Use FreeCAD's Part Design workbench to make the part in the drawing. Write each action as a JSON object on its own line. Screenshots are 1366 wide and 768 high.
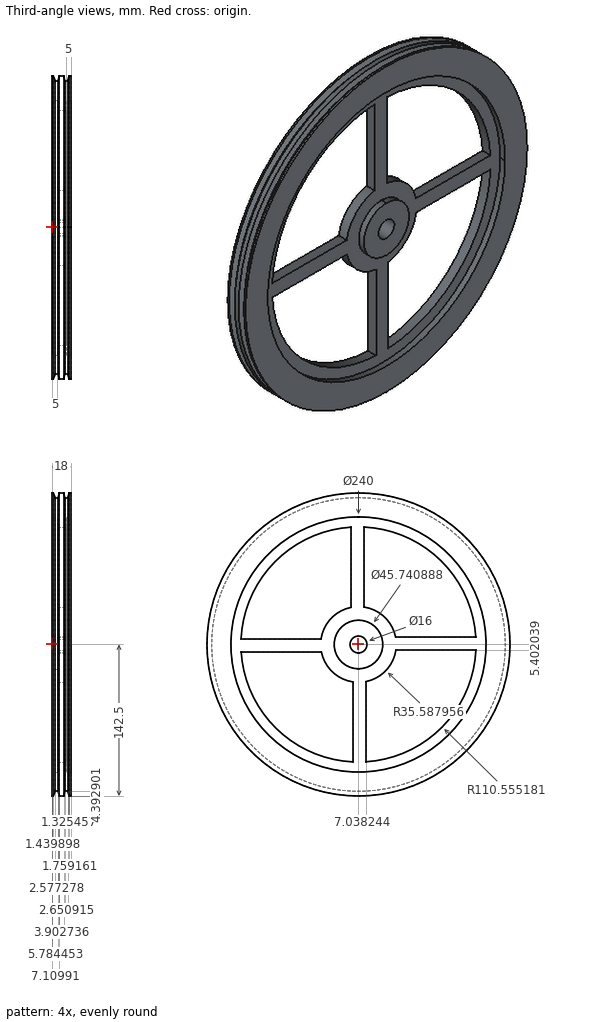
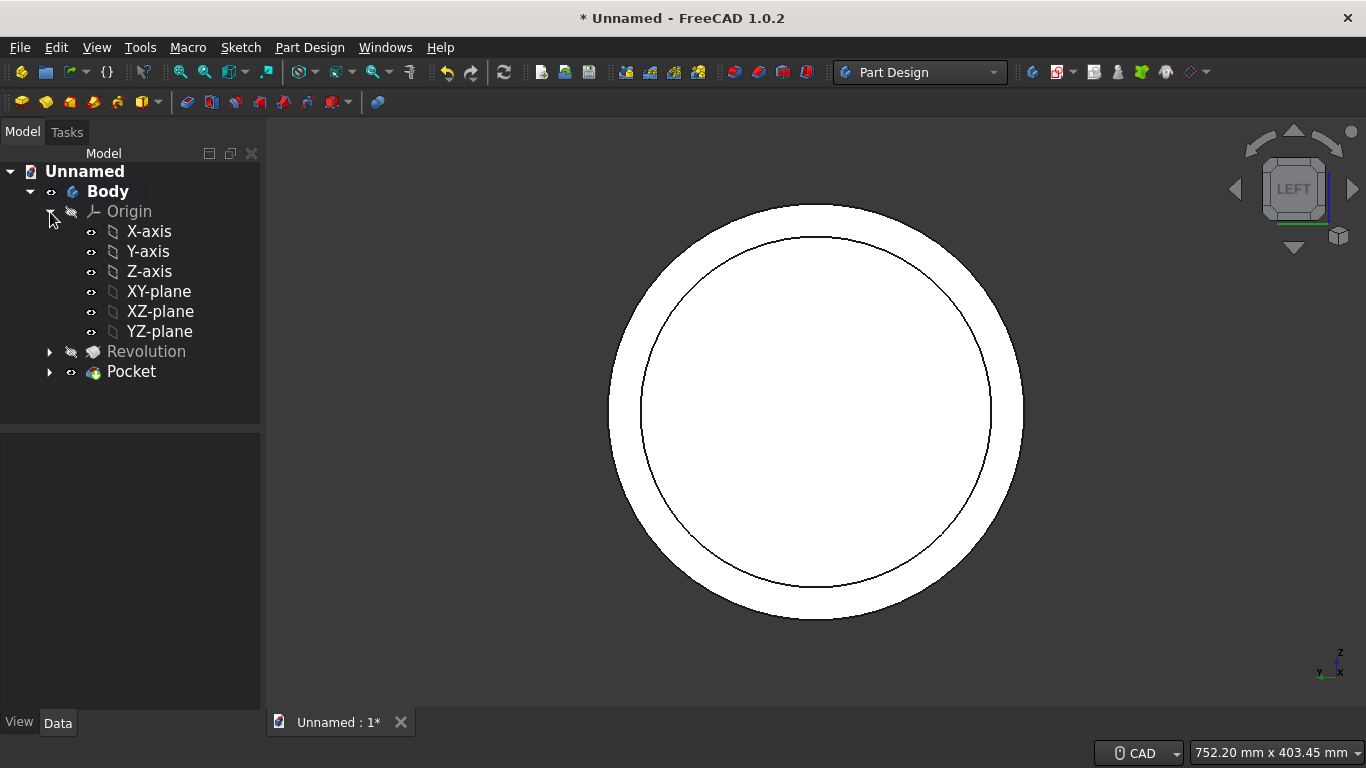
{"action": "left_click", "coordinate": [136, 332]}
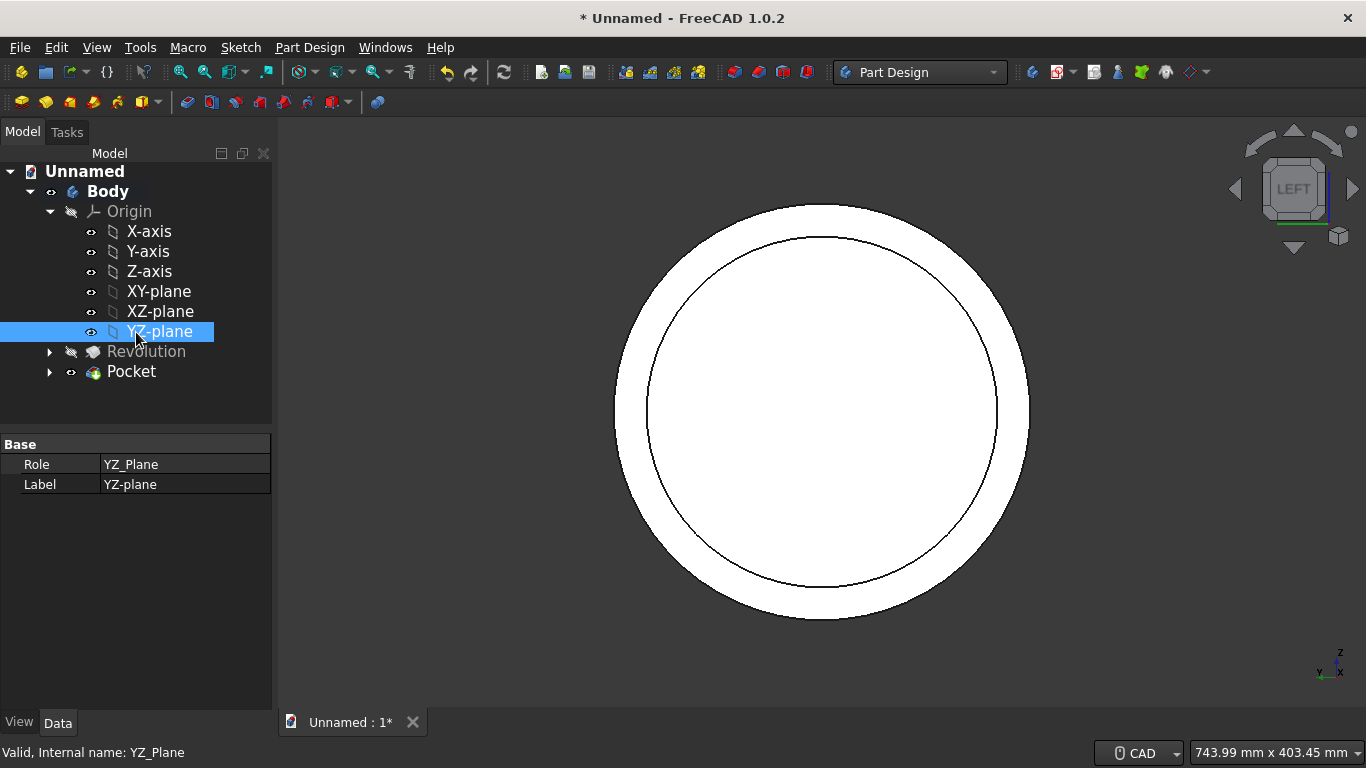
{"action": "left_click", "coordinate": [1190, 72]}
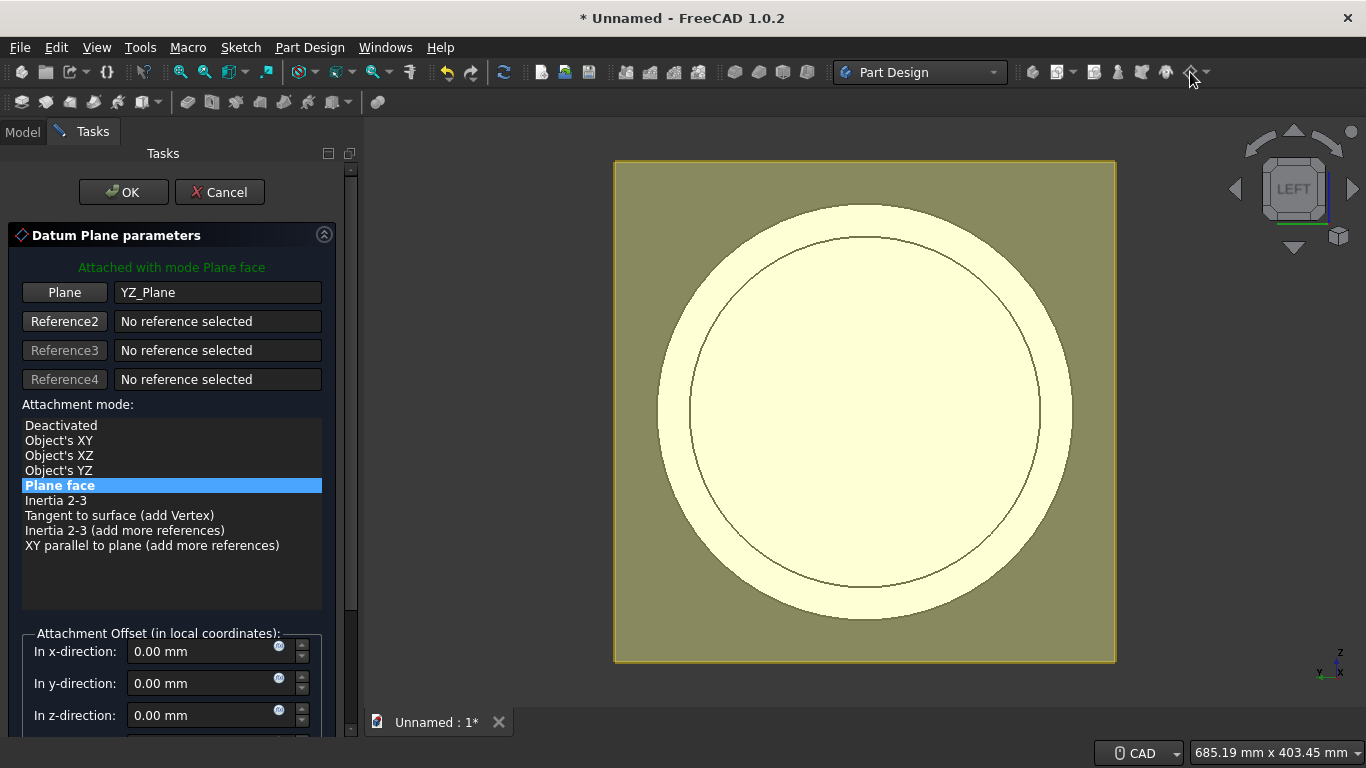
{"action": "triple_click", "coordinate": [210, 715]}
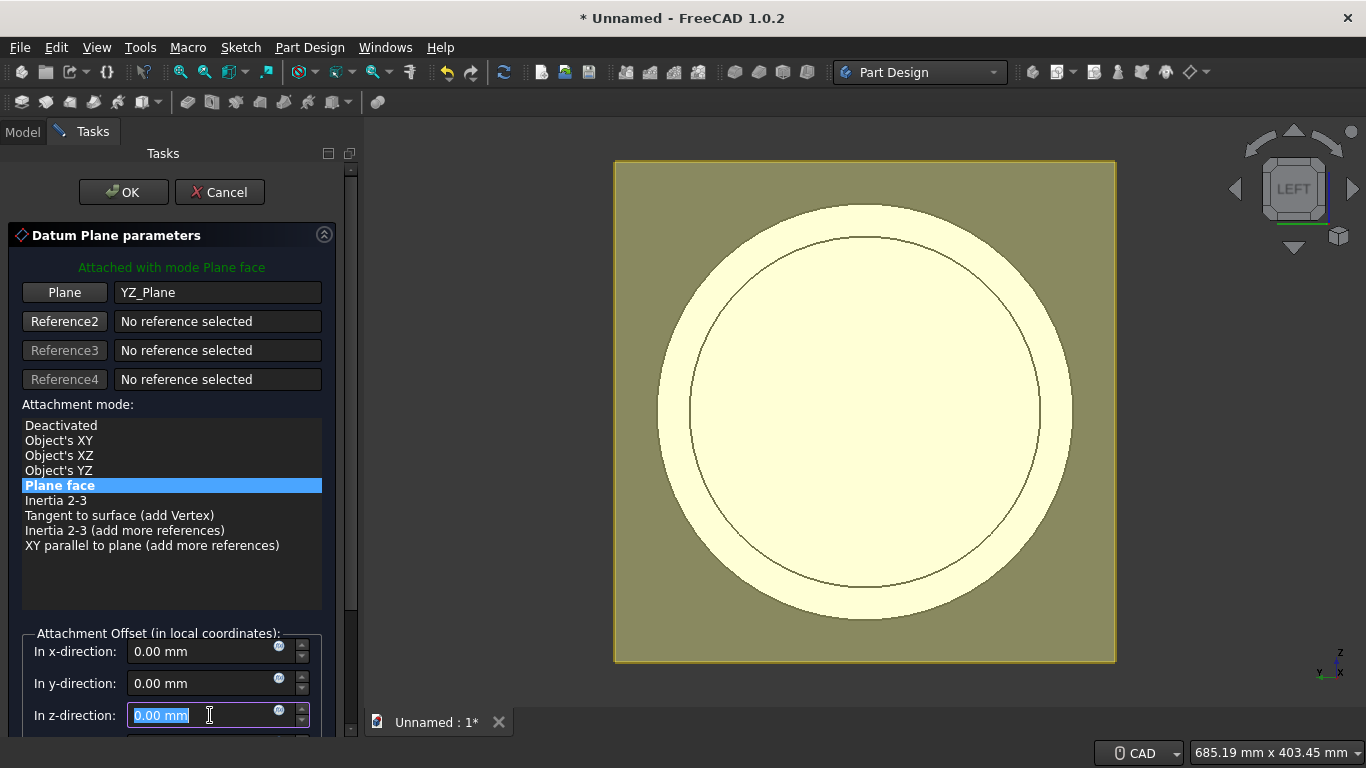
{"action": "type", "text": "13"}
{"action": "key", "text": "Tab"}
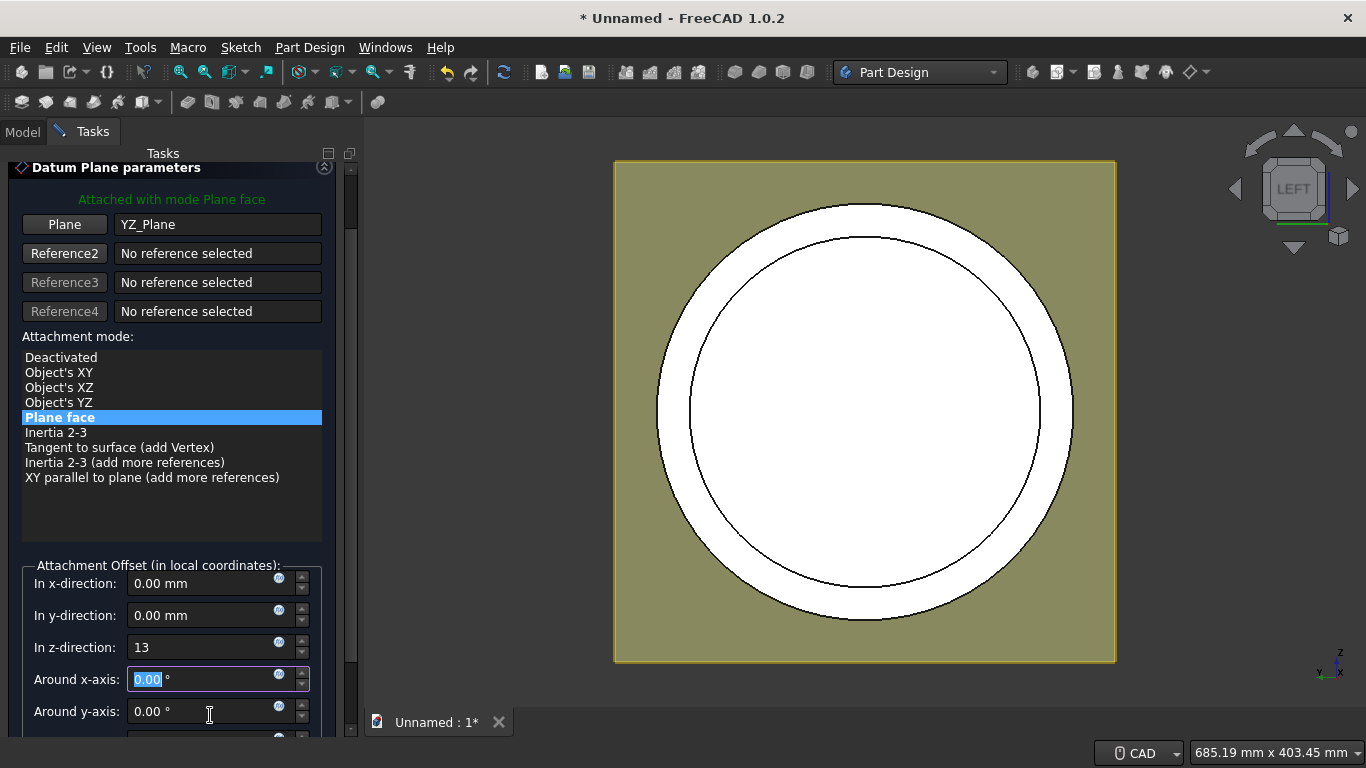
{"action": "scroll", "coordinate": [351, 450], "scroll_direction": "up", "scroll_amount": 2}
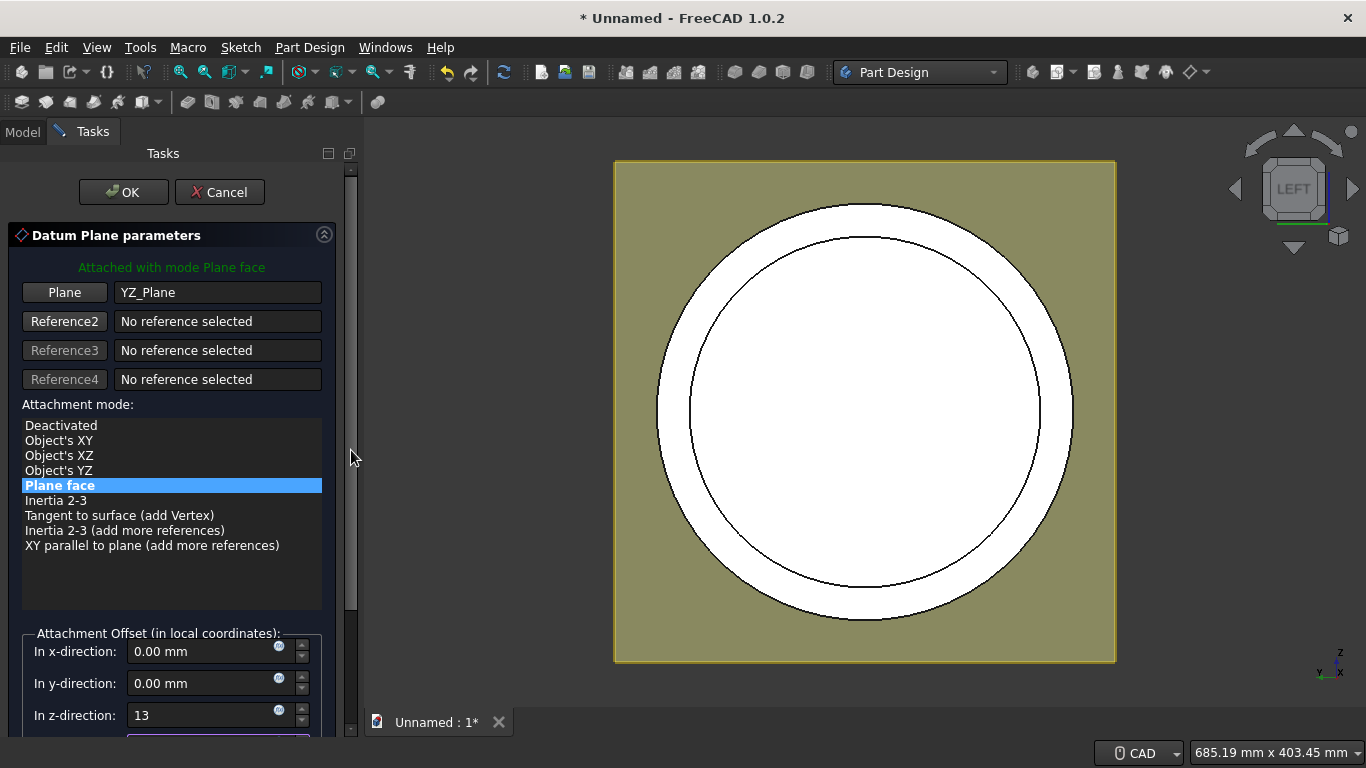
{"action": "left_click", "coordinate": [124, 192]}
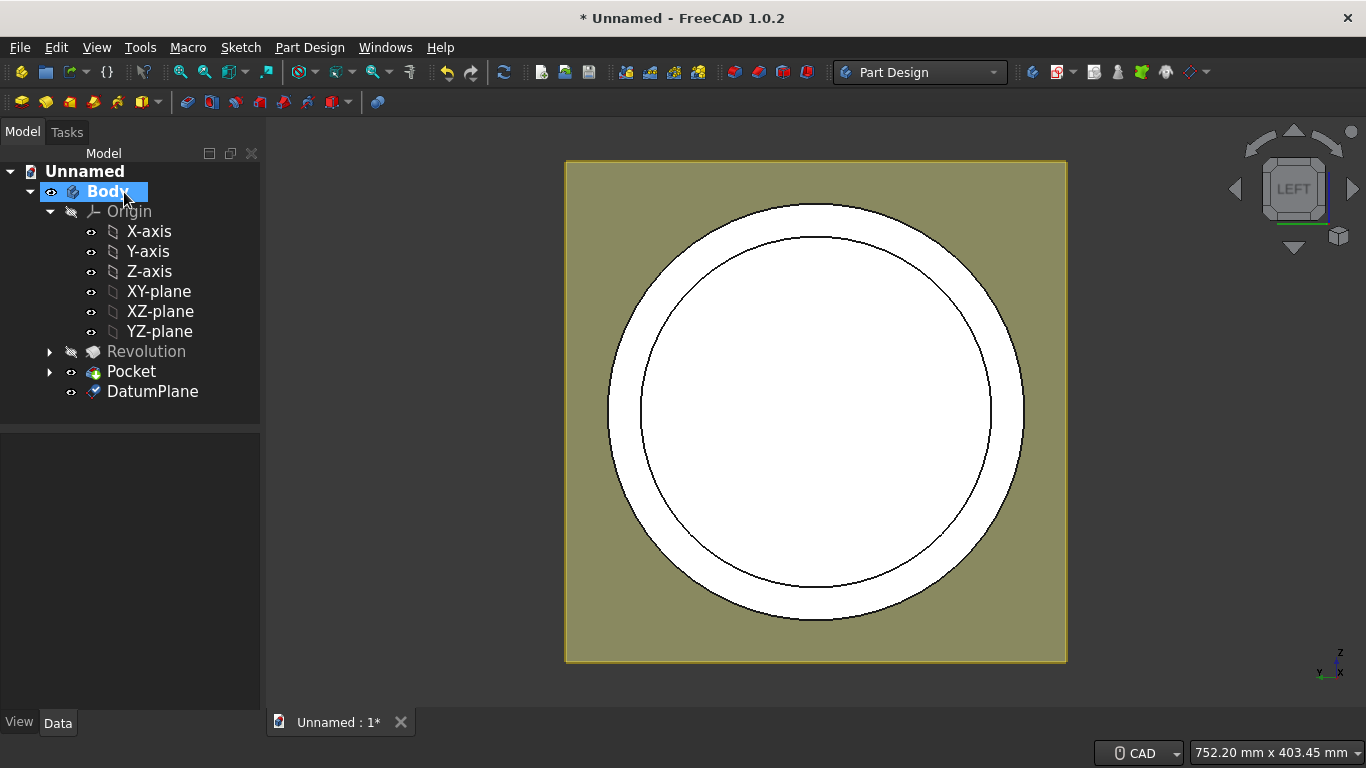
{"action": "left_click", "coordinate": [116, 392]}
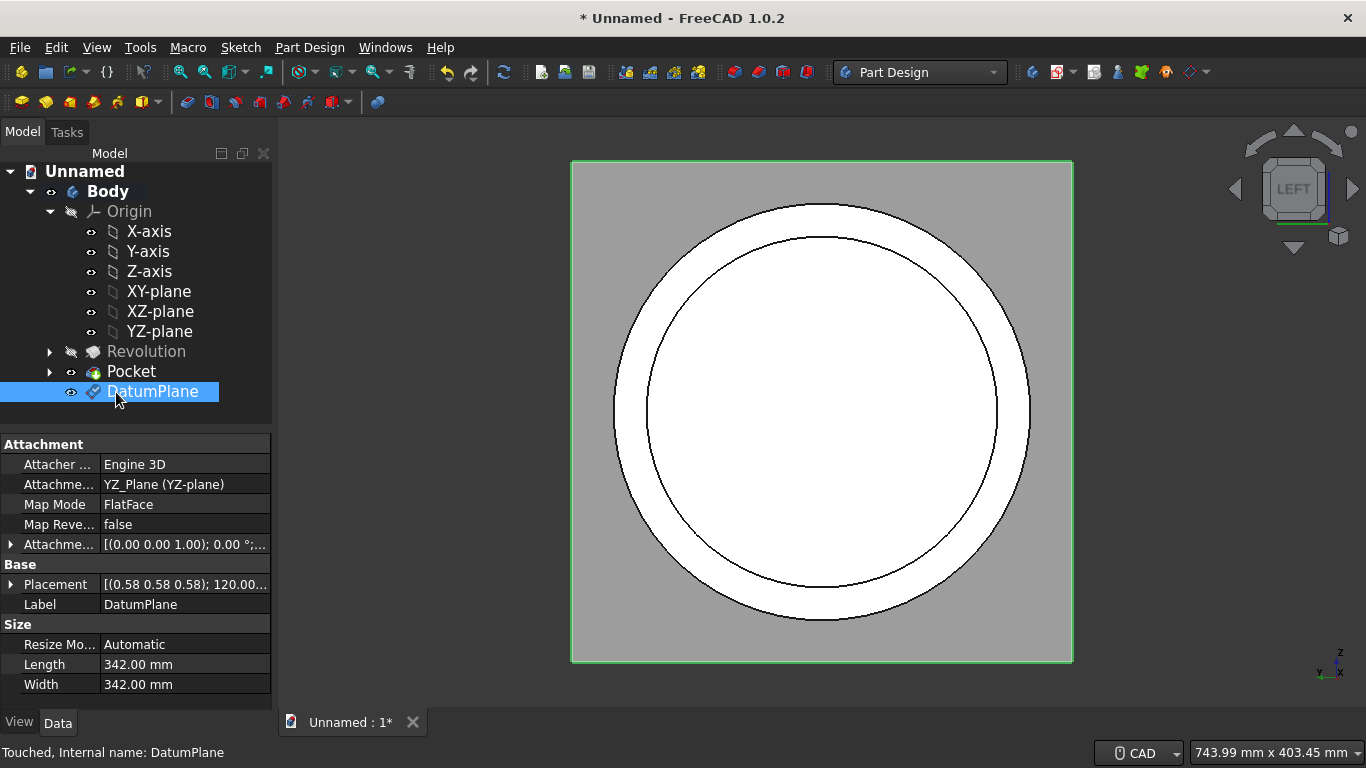
{"action": "left_click", "coordinate": [1058, 72]}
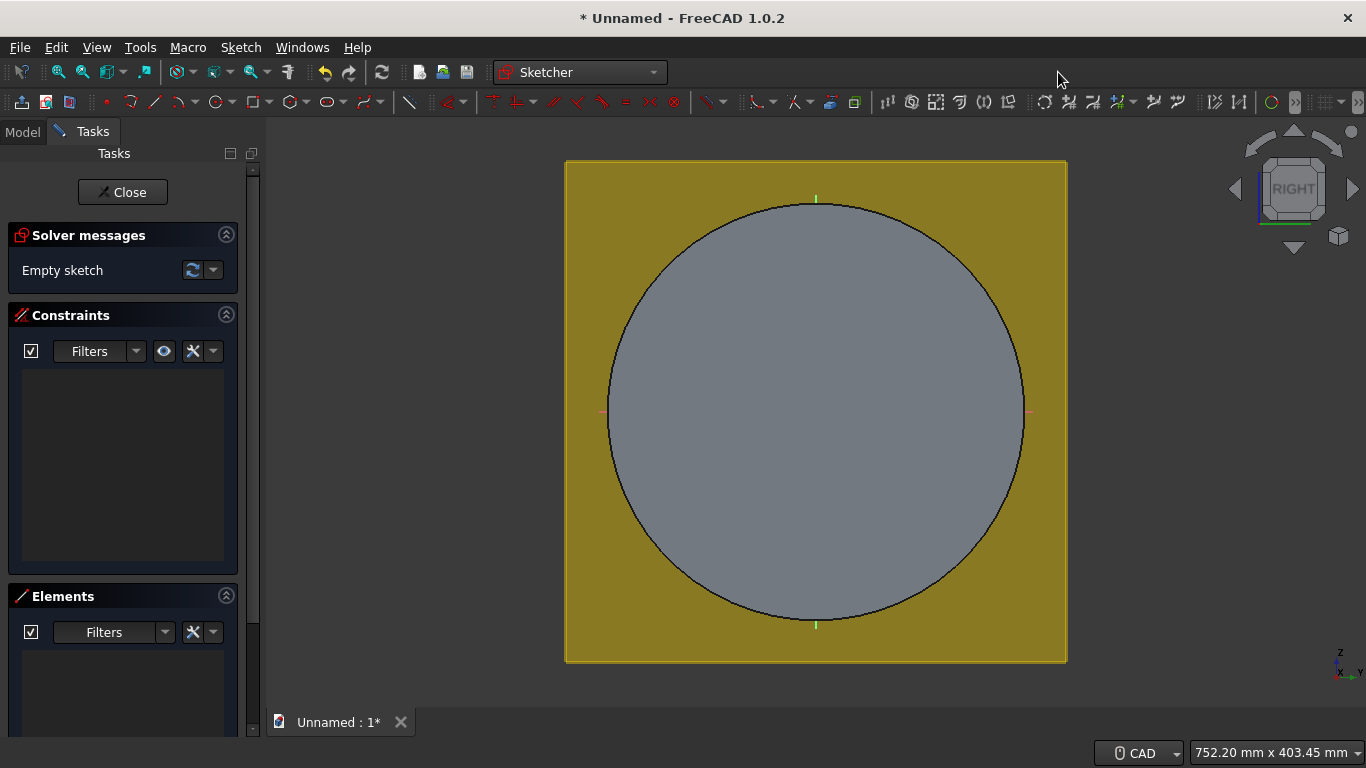
{"action": "key", "text": "q s"}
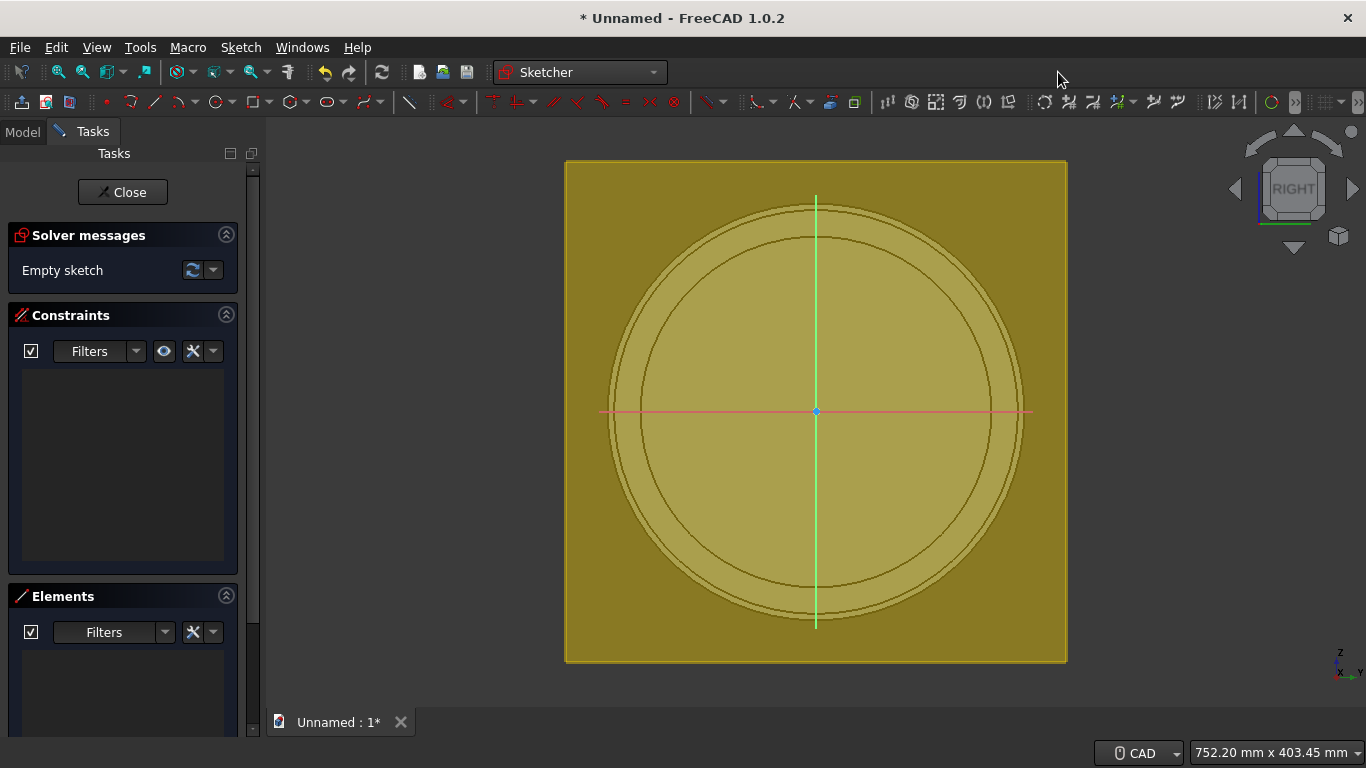
{"action": "key", "text": "g c"}